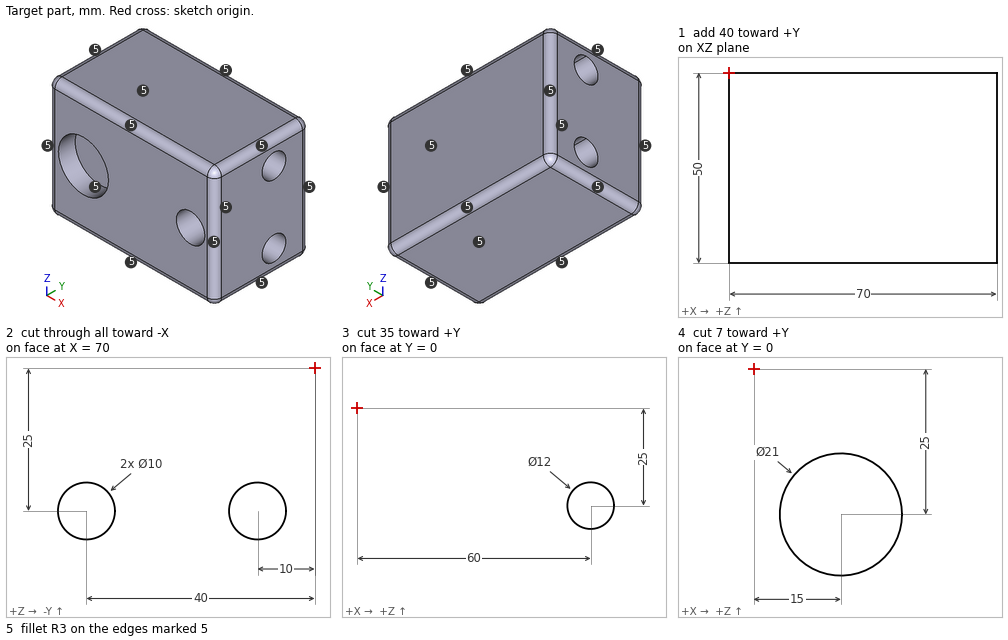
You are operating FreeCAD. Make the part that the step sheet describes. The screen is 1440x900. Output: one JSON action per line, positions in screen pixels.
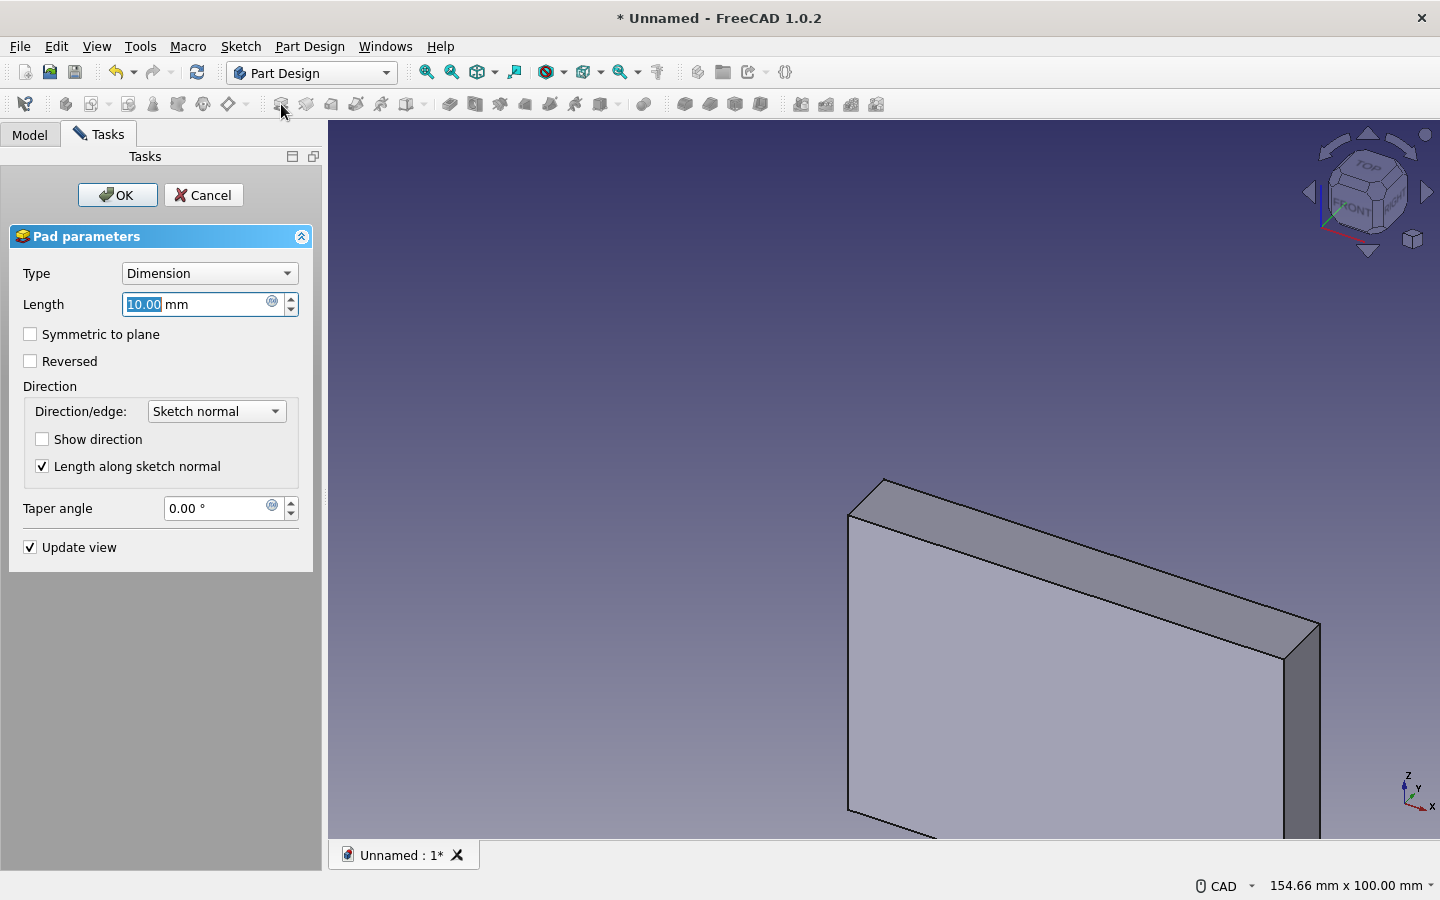
{"action": "type", "text": "40"}
{"action": "key", "text": "Tab"}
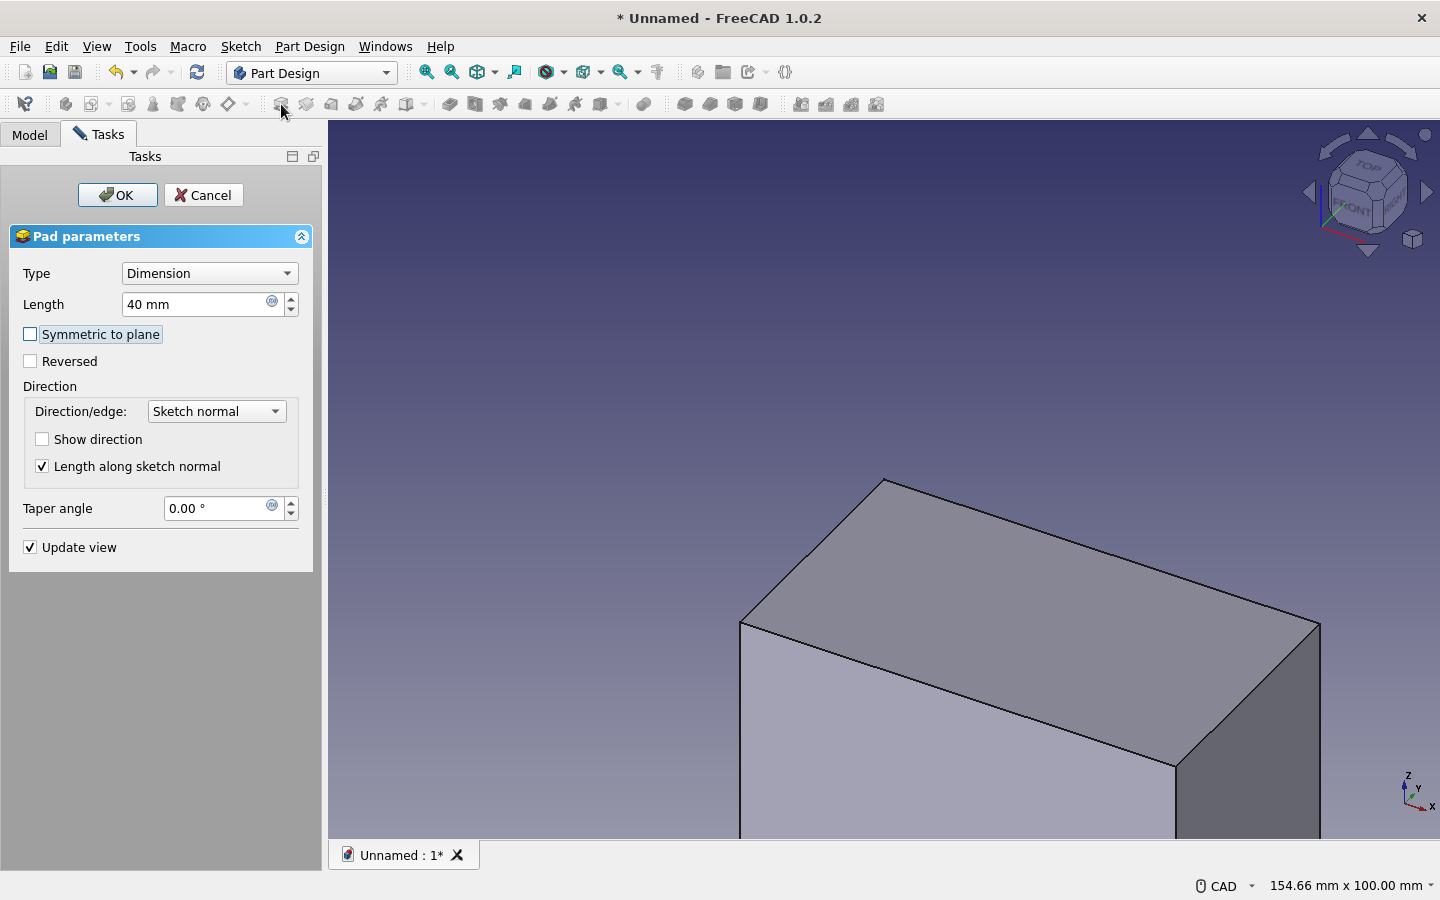
{"action": "left_click", "coordinate": [31, 361]}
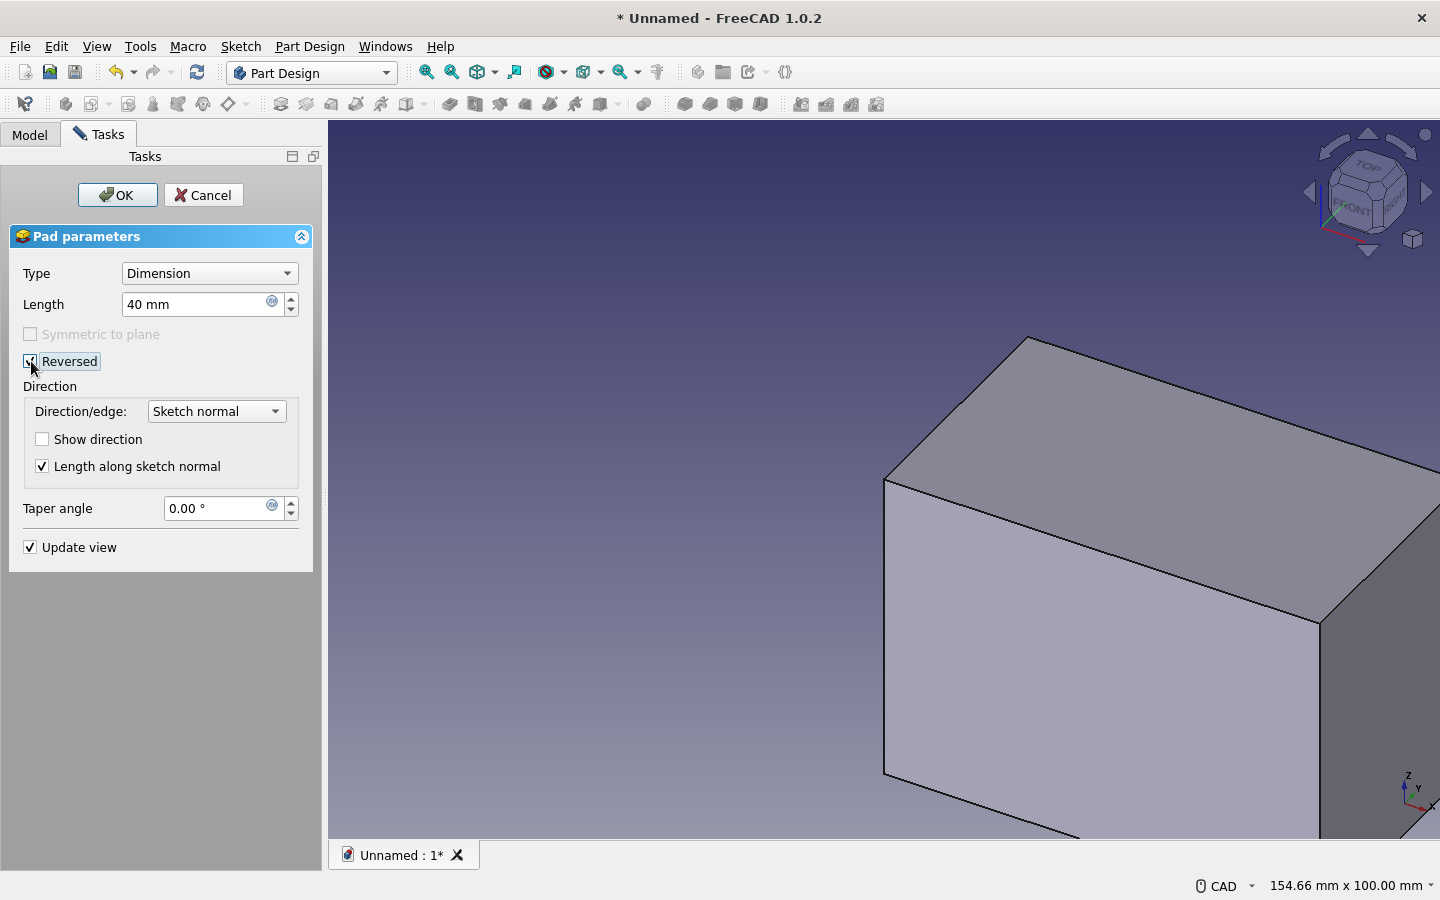
{"action": "left_click", "coordinate": [118, 195]}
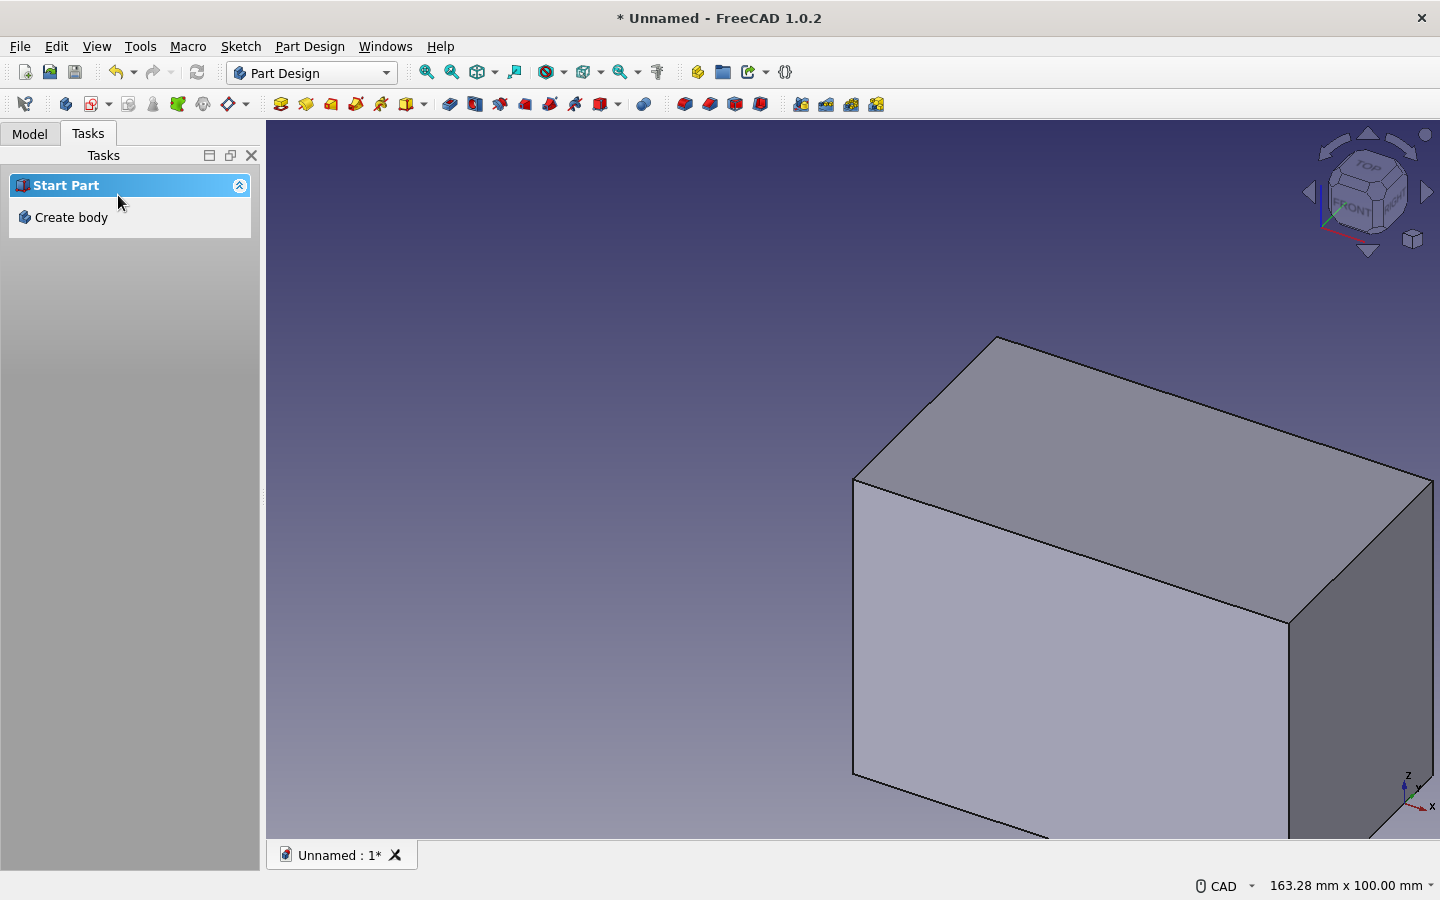
{"action": "key", "text": "v f"}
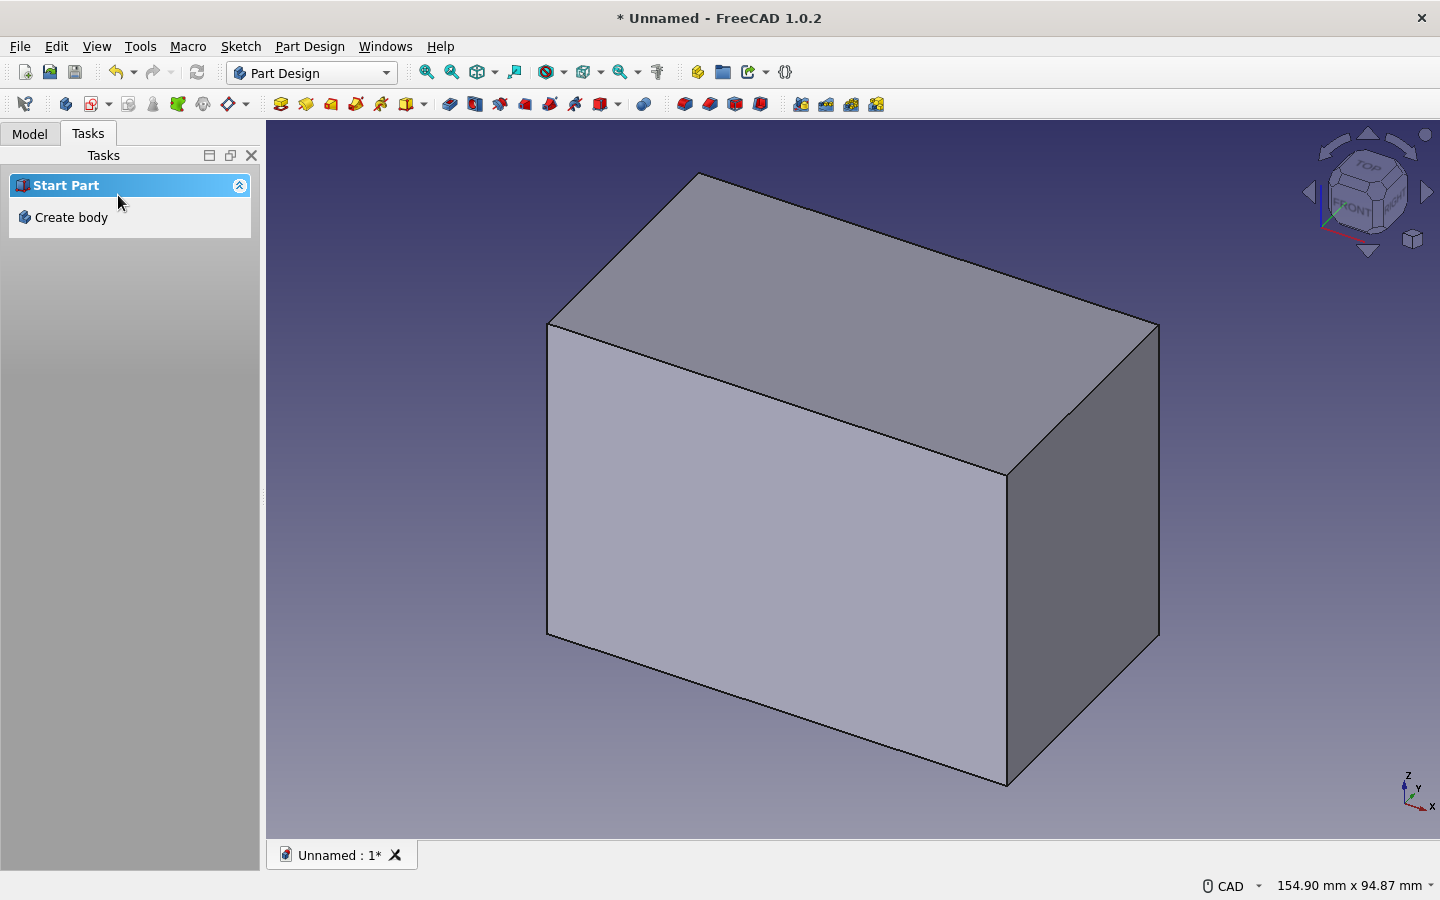
{"action": "left_click", "coordinate": [1083, 555]}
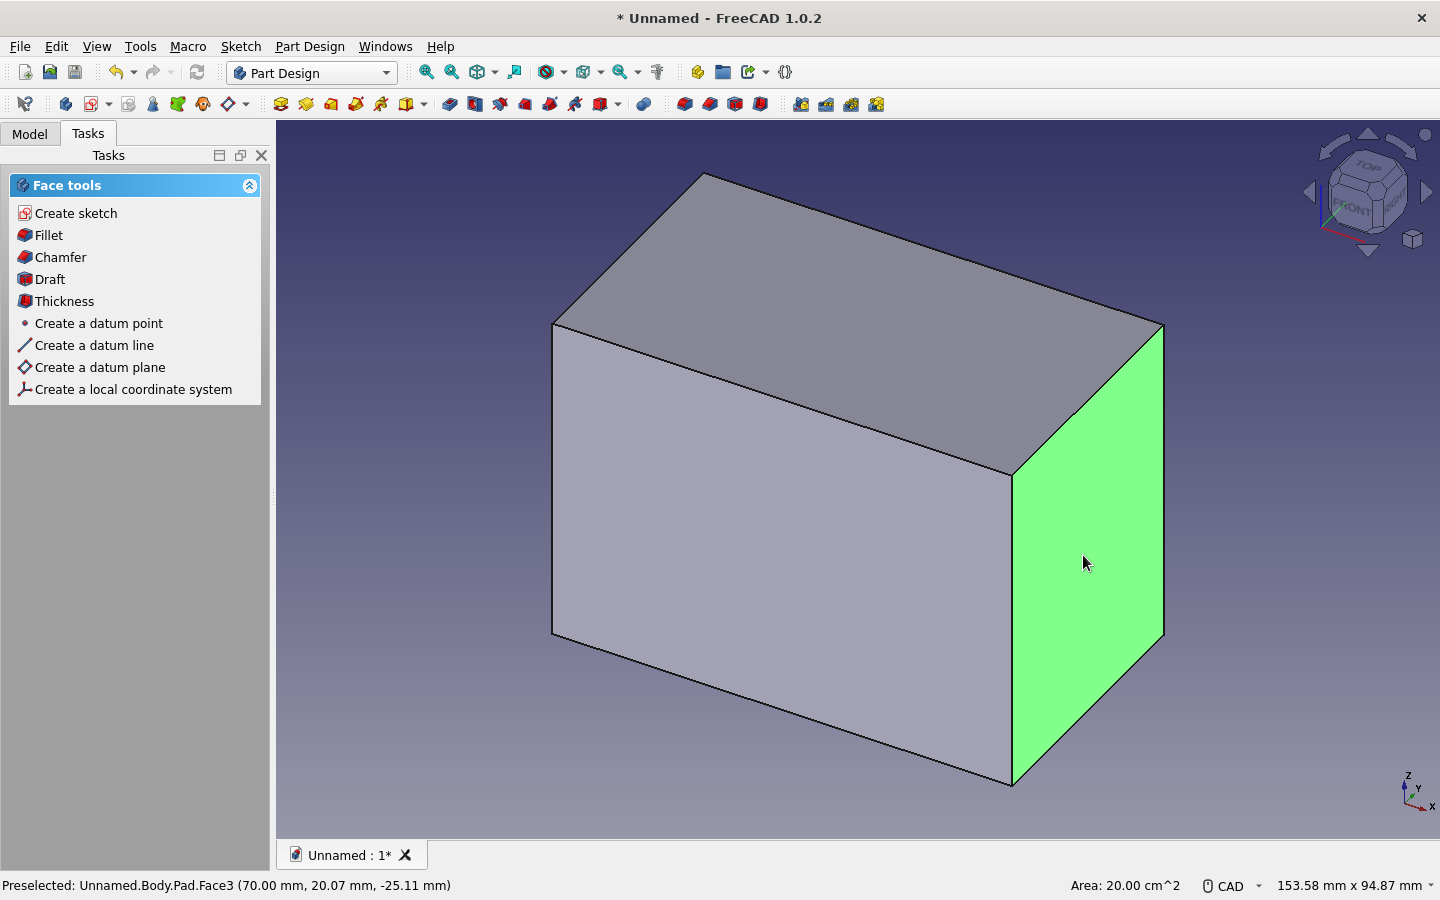
{"action": "left_click", "coordinate": [90, 104]}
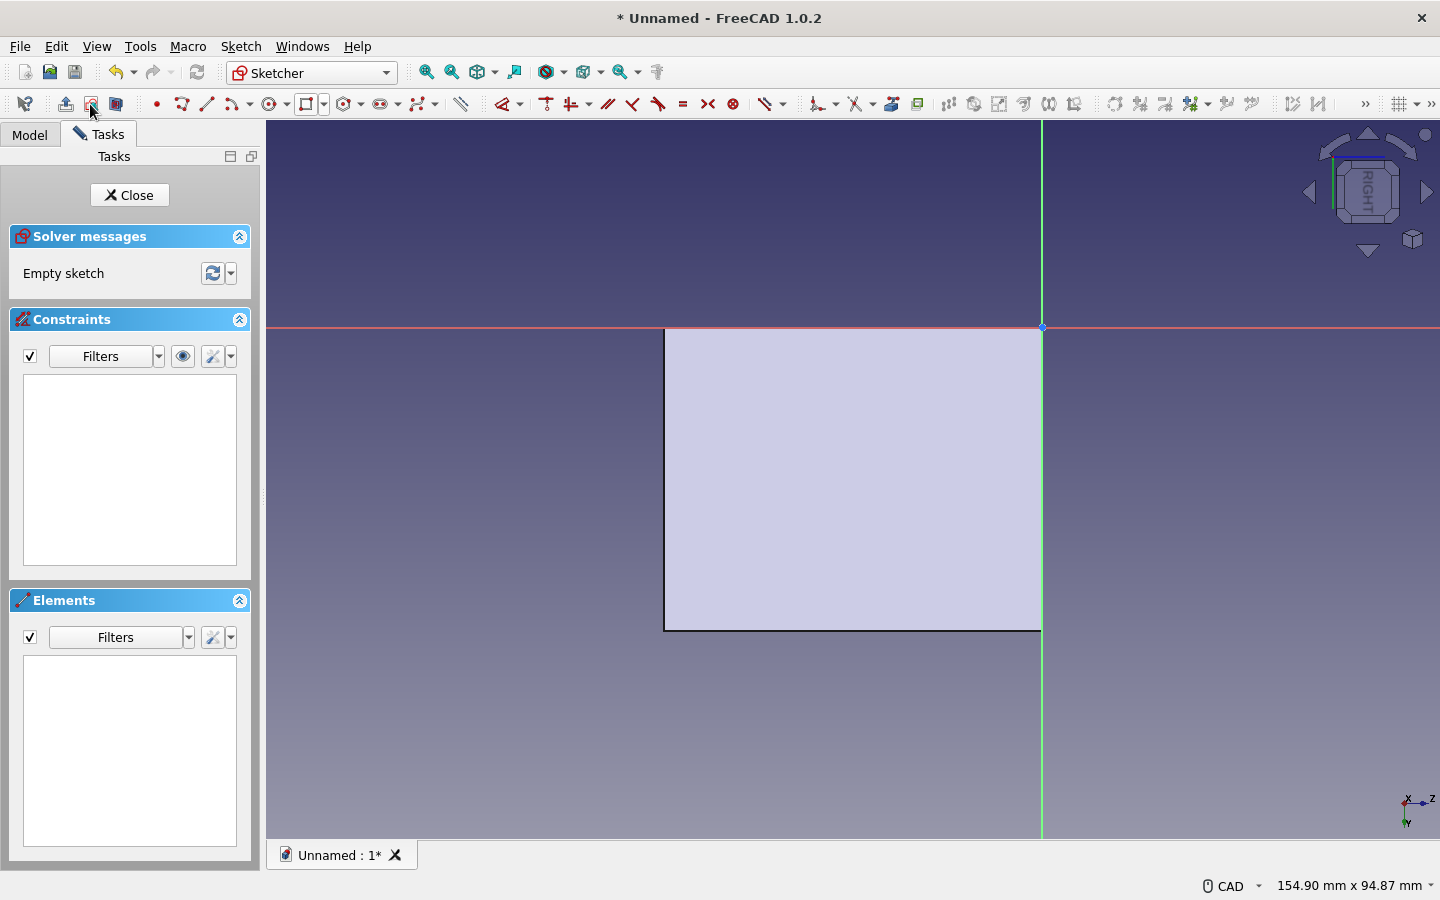
{"action": "scroll", "coordinate": [943, 411], "scroll_direction": "up", "scroll_amount": 4}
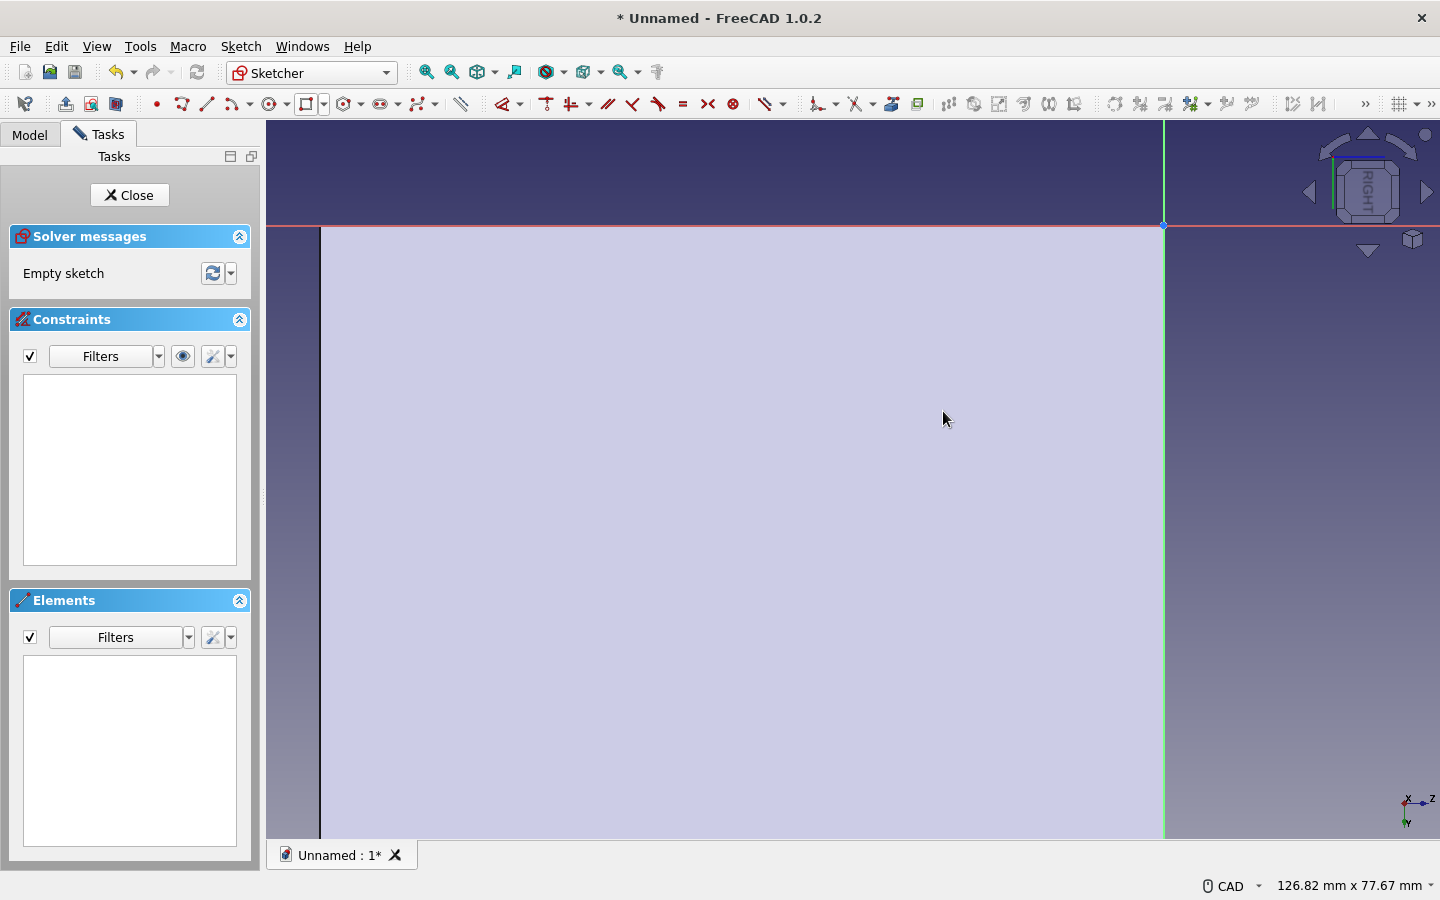
{"action": "key", "text": "g c"}